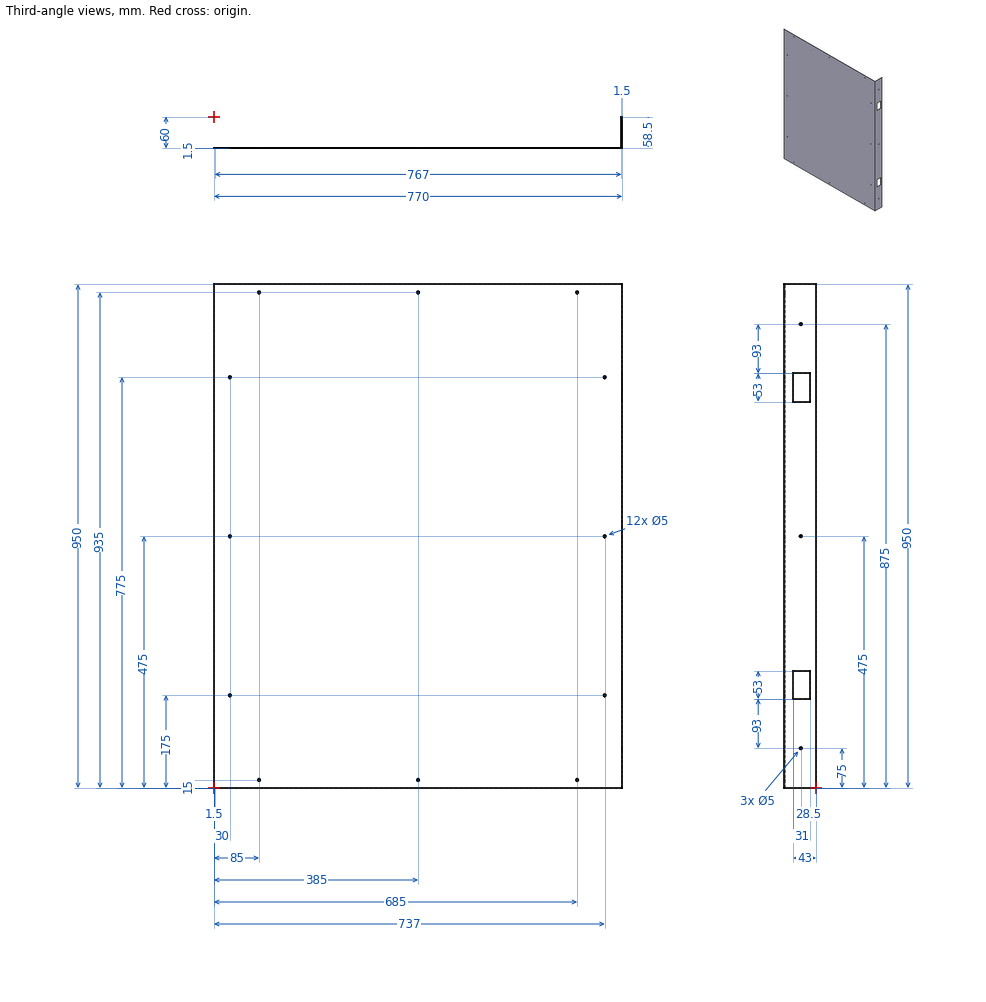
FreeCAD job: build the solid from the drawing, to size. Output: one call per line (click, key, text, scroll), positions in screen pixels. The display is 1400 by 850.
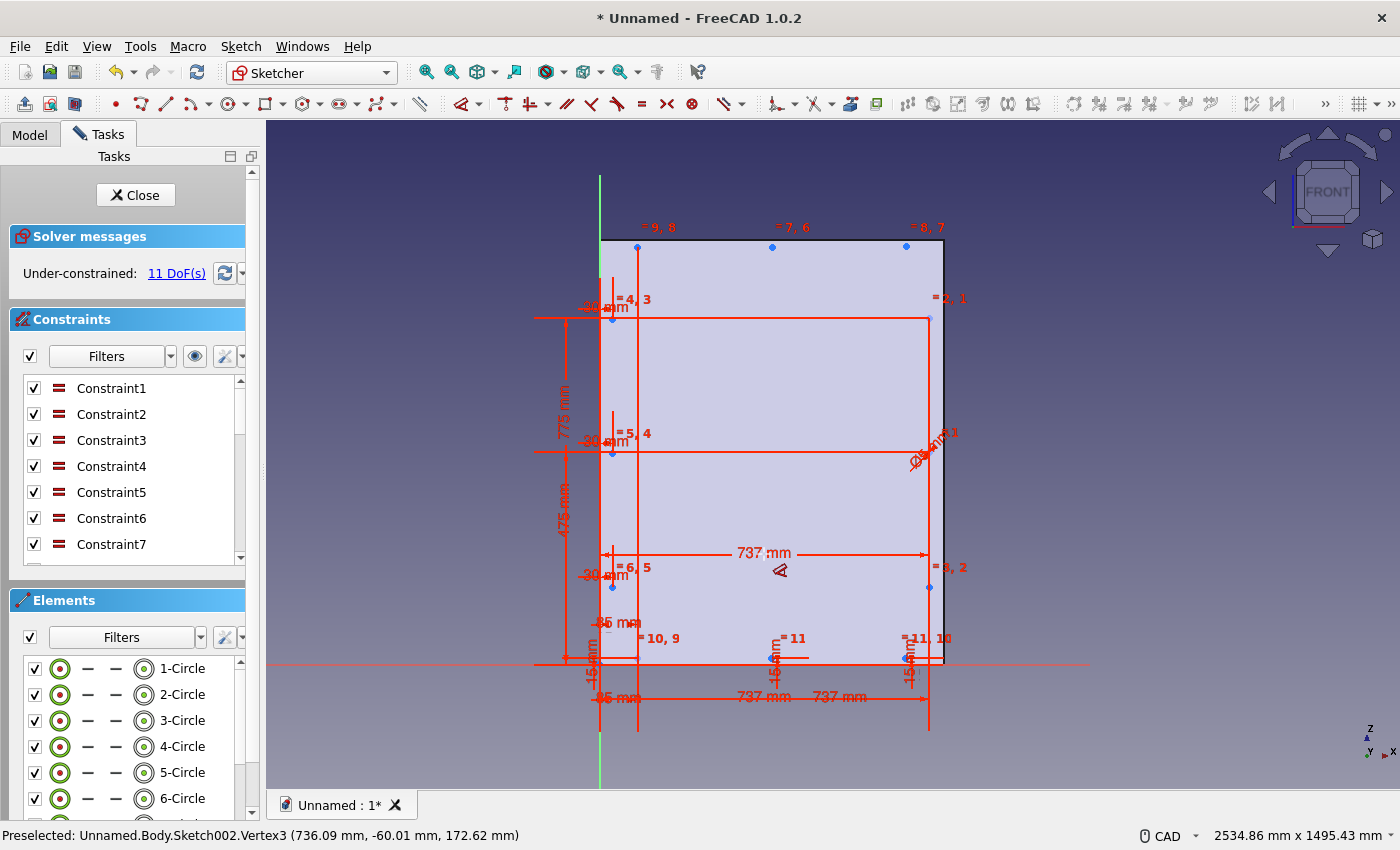
click(929, 588)
click(566, 599)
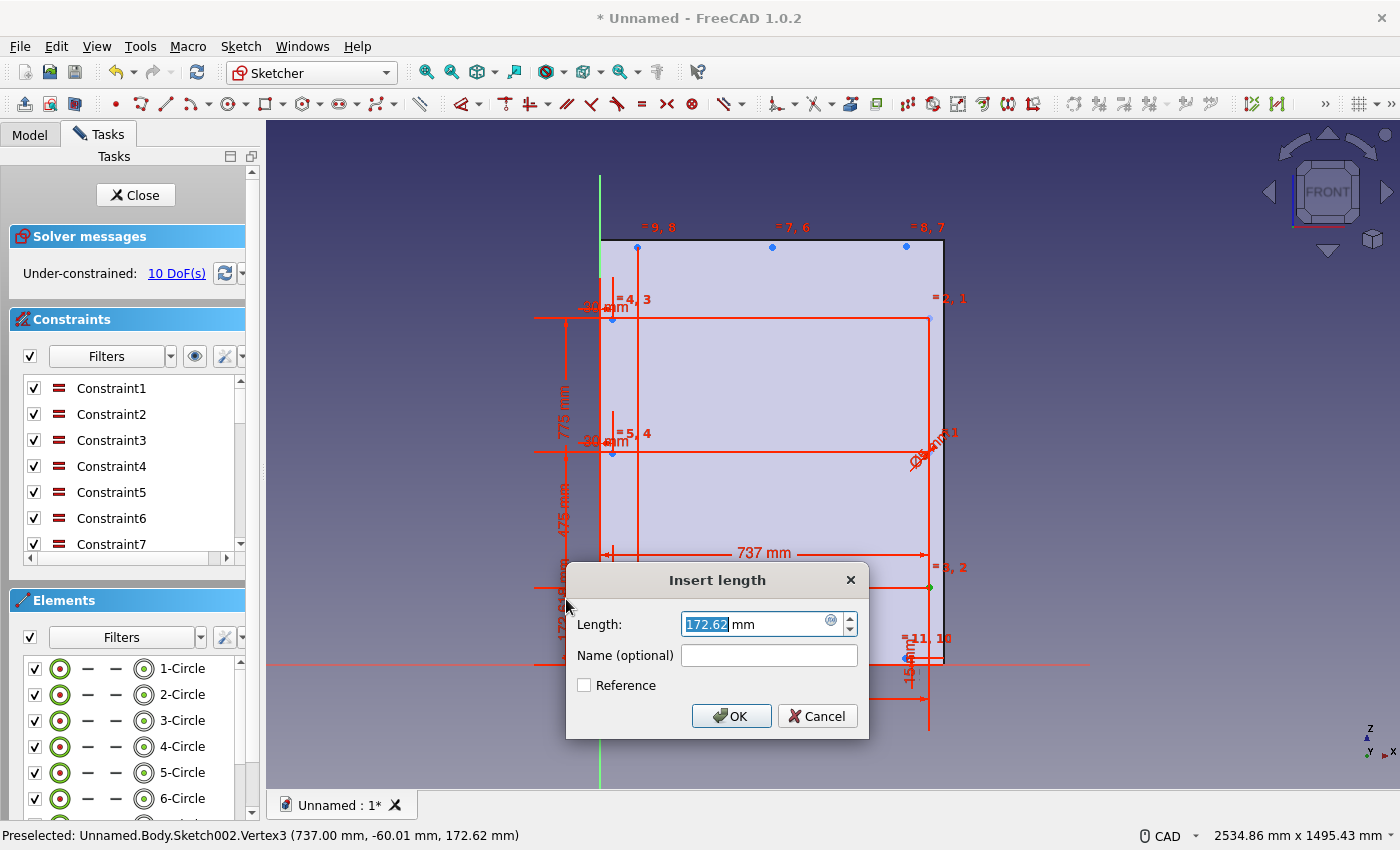
text(175)
key(Return)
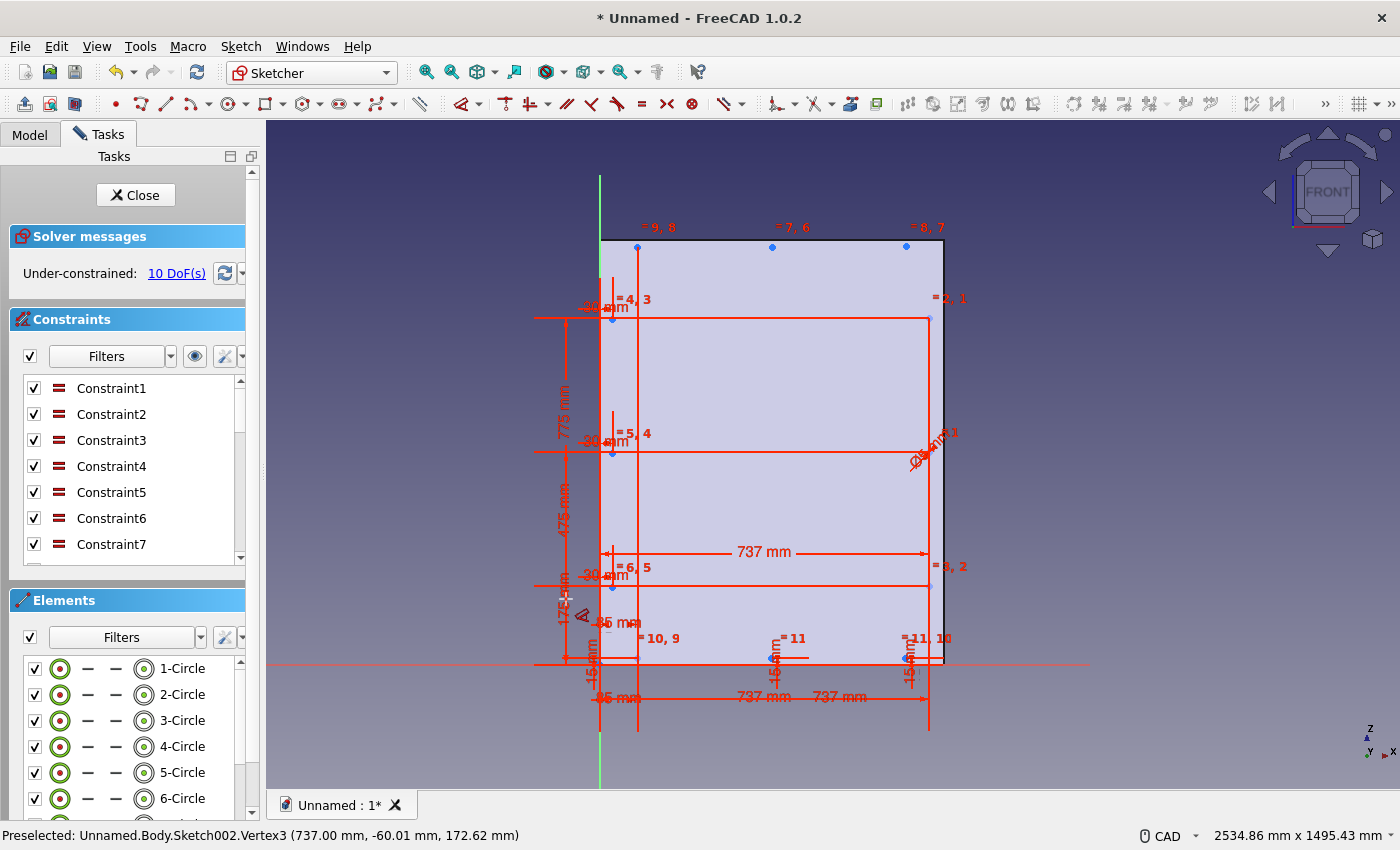
click(613, 319)
click(566, 371)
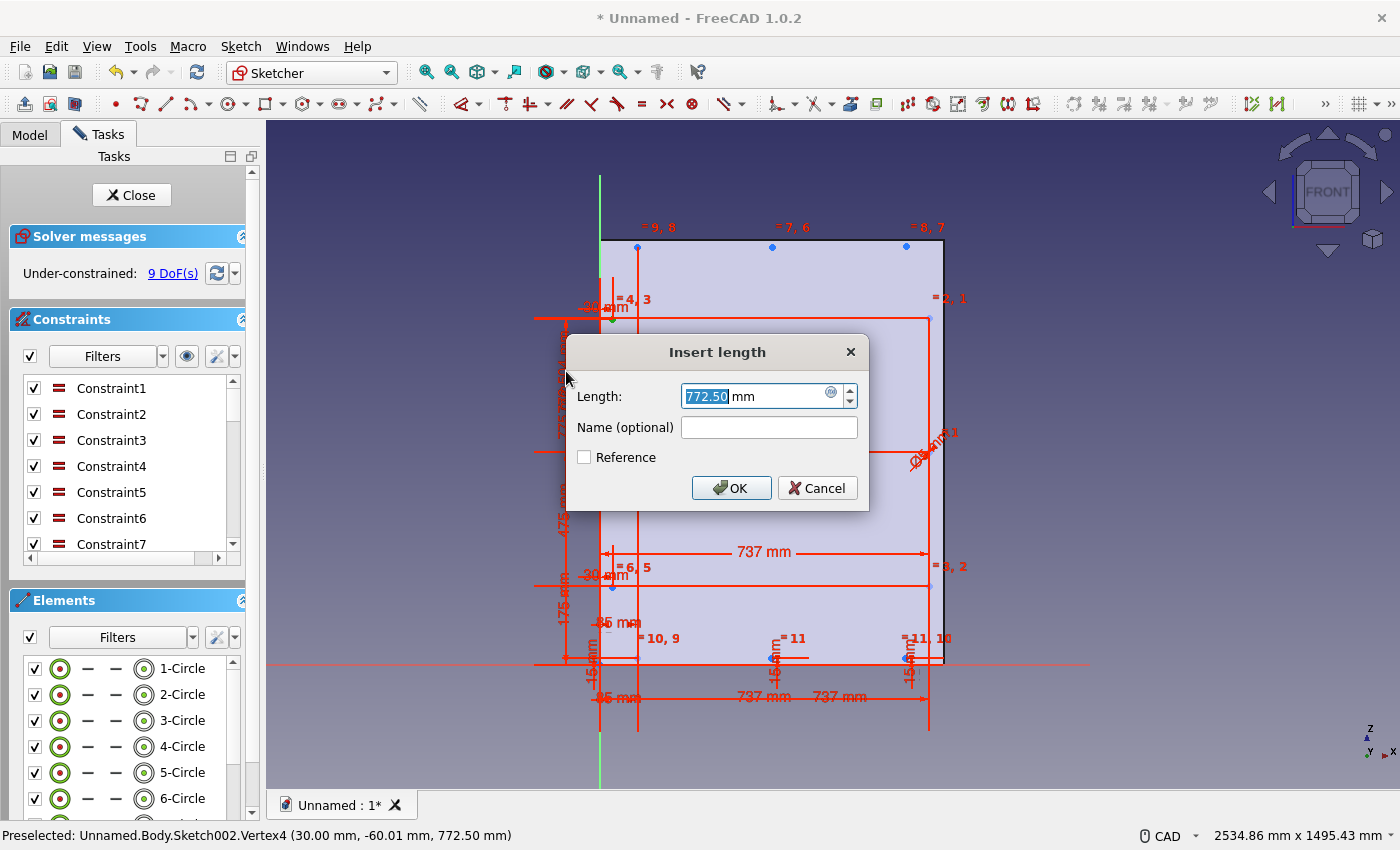
text(775)
key(Return)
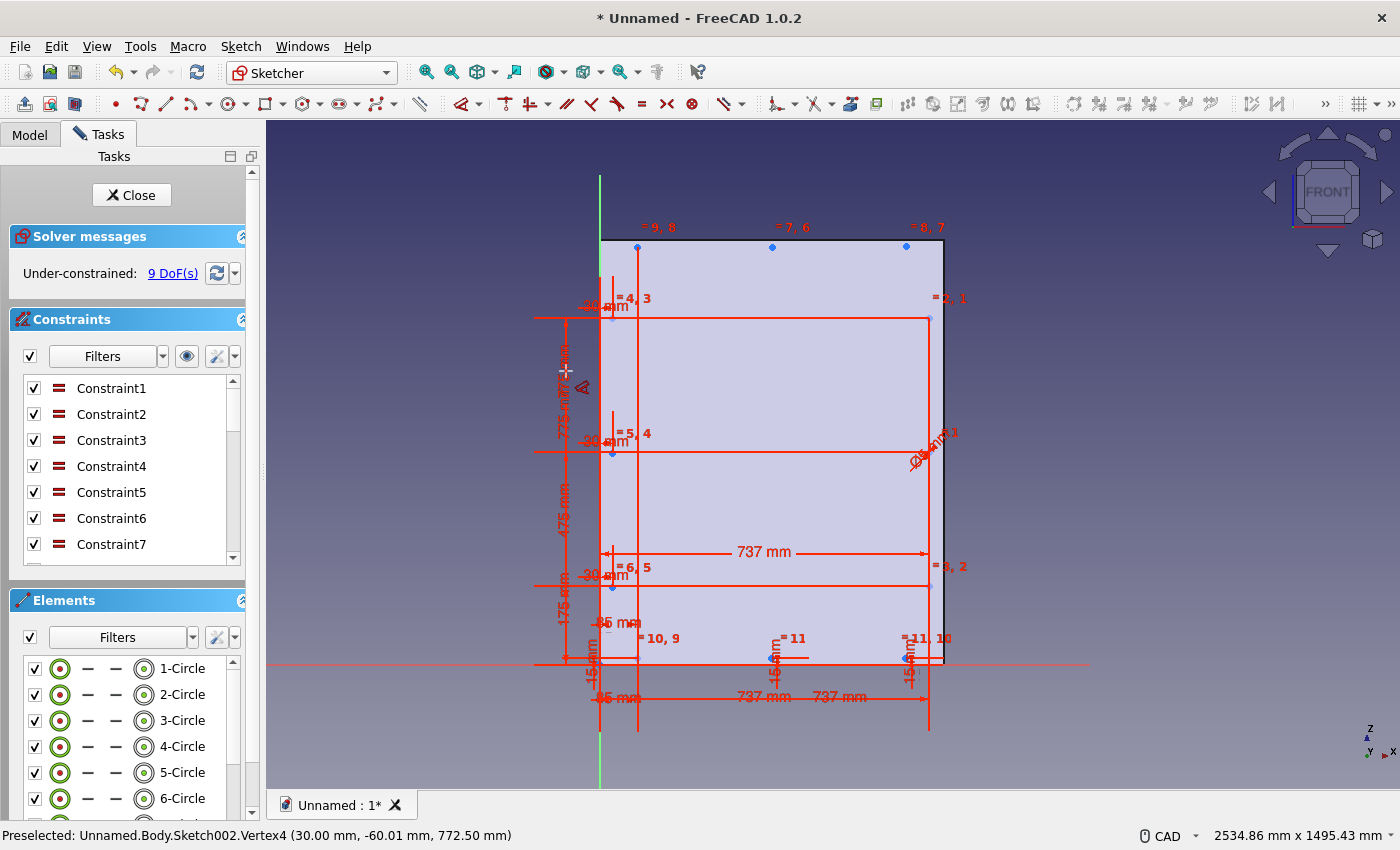
click(613, 453)
click(566, 485)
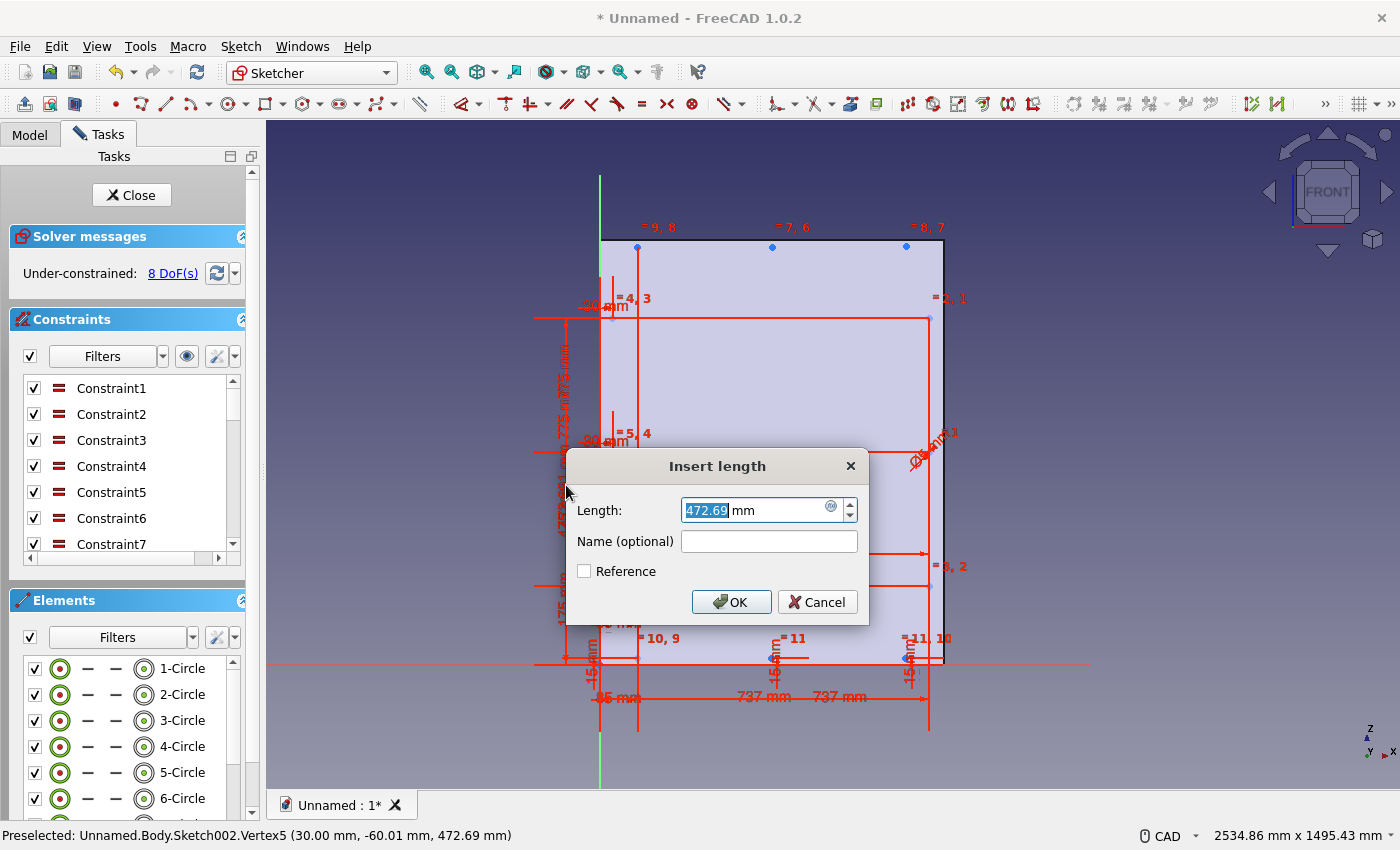
text(475)
key(Return)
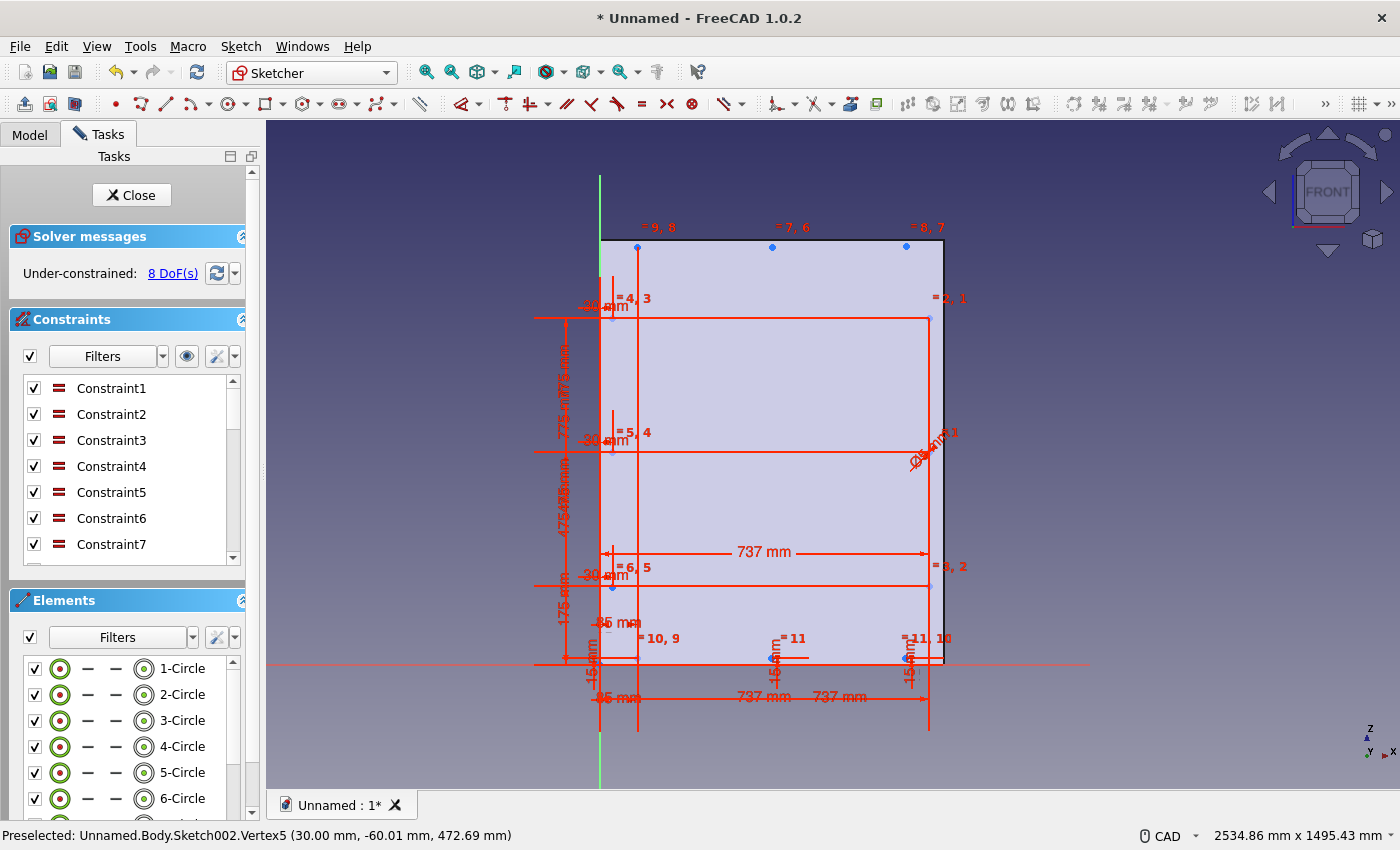
click(613, 587)
click(647, 599)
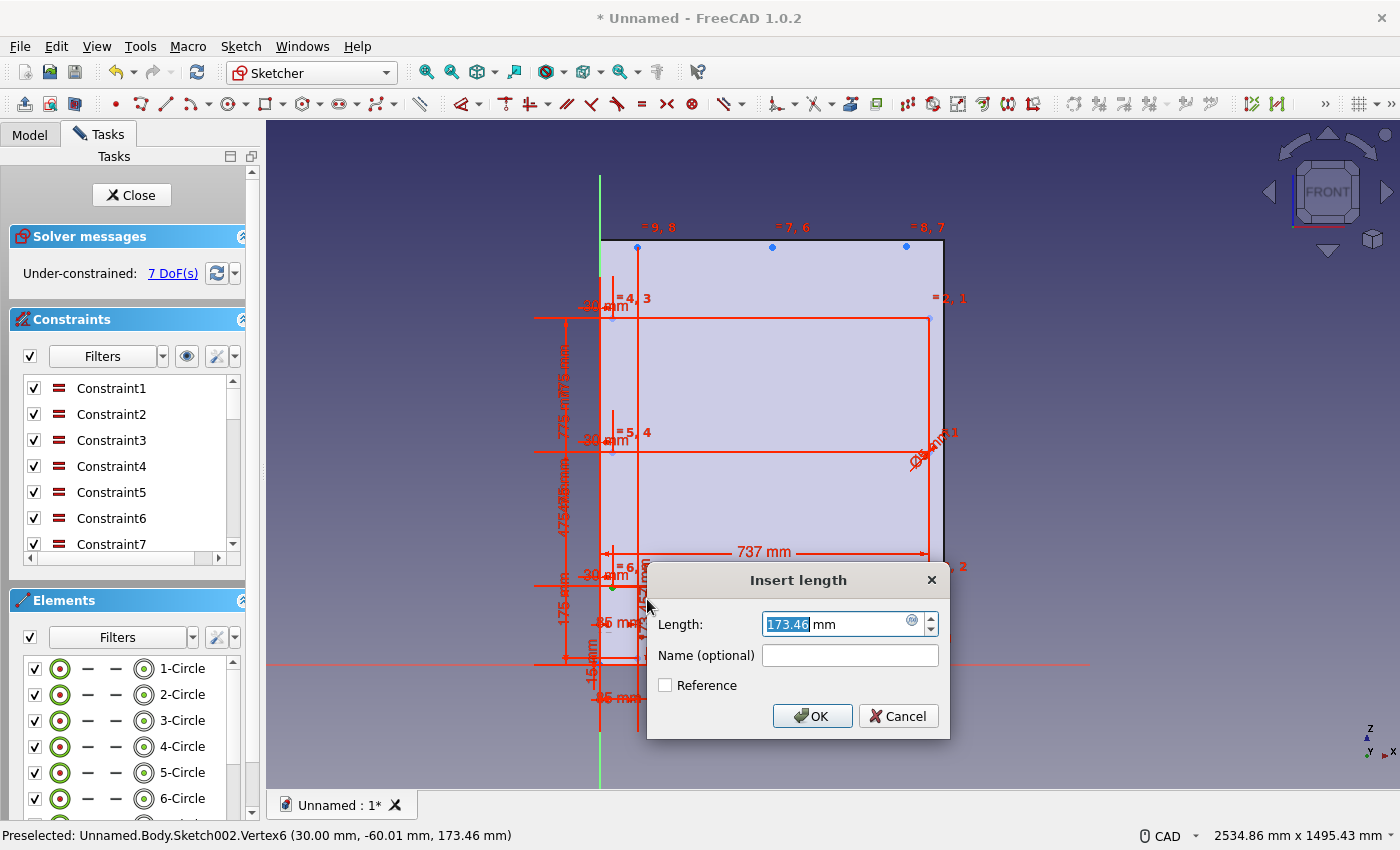
text(175)
key(Return)